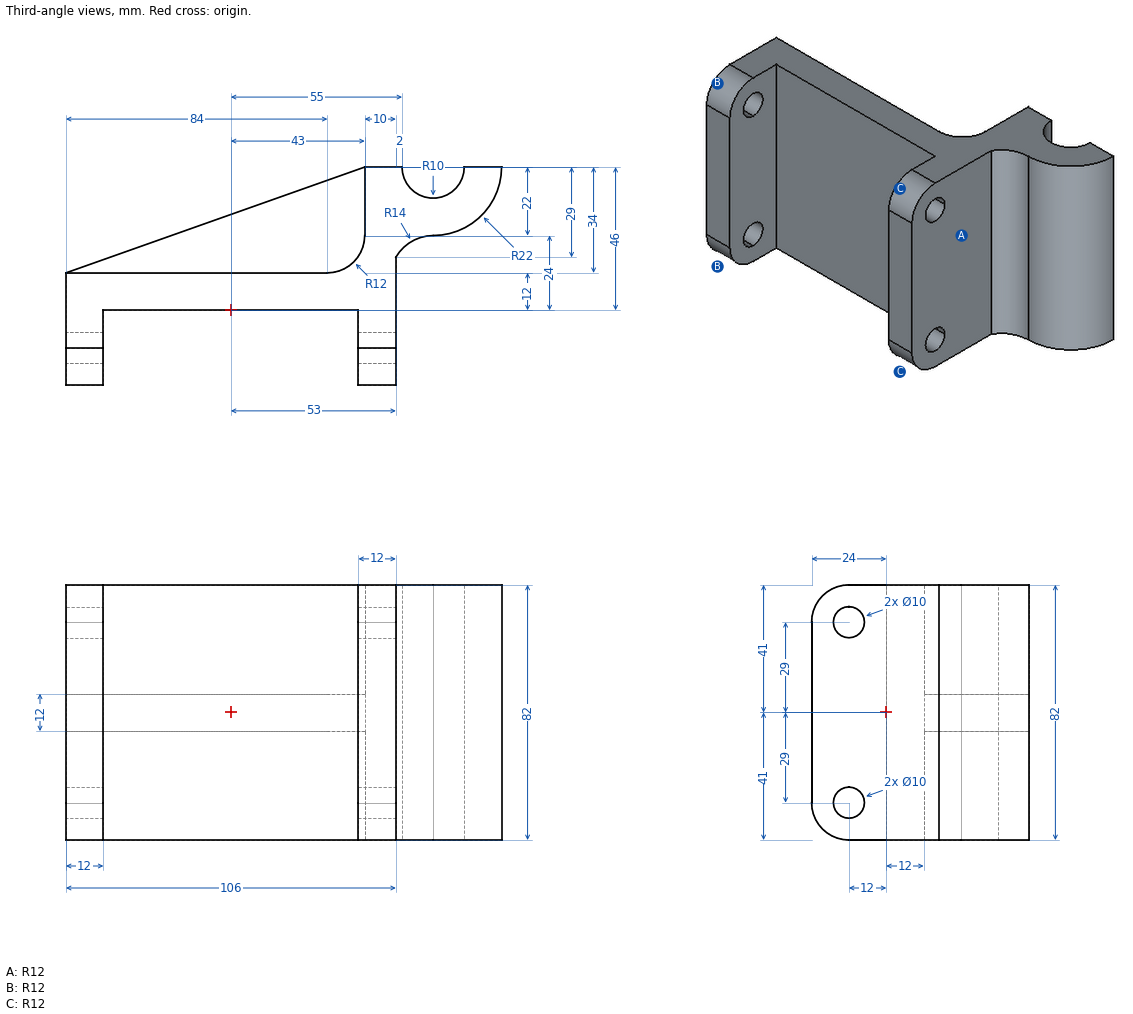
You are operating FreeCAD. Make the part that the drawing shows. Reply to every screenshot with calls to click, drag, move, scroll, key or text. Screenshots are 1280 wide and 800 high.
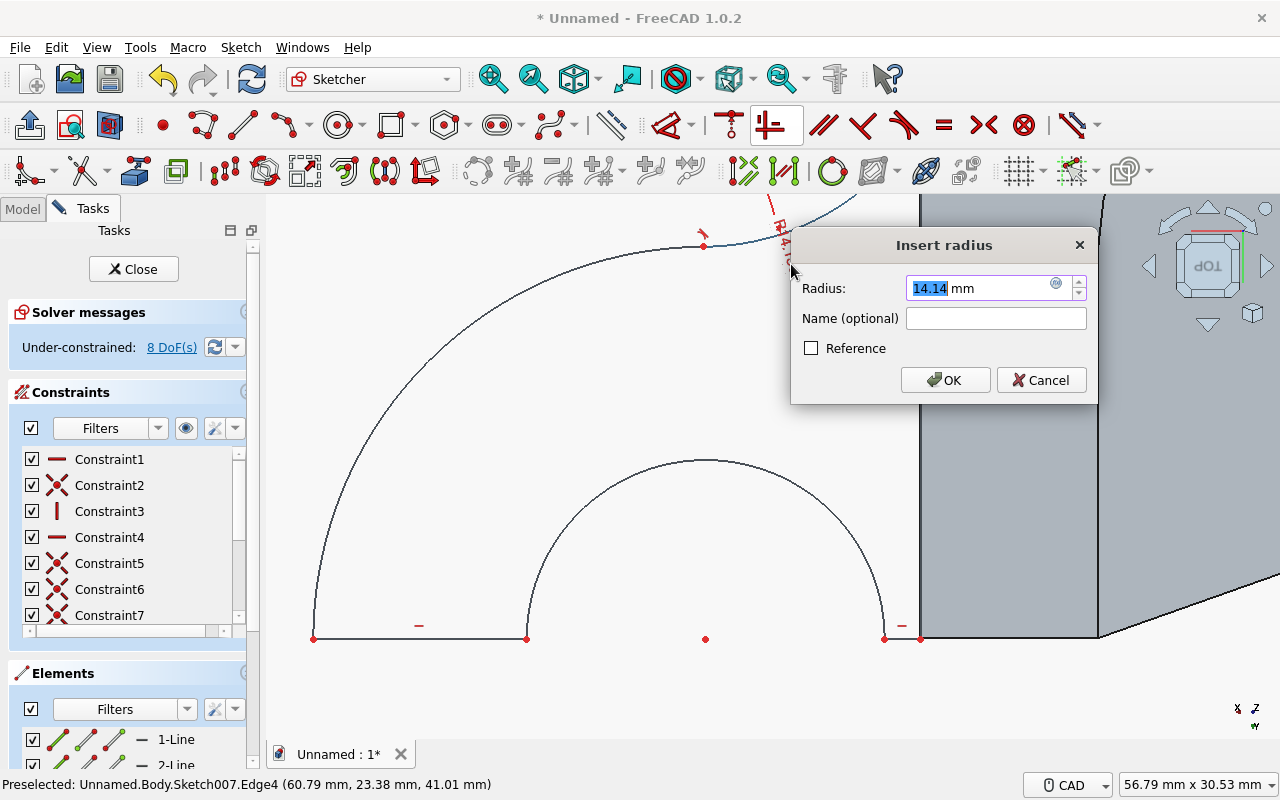
text(14)
key(Return)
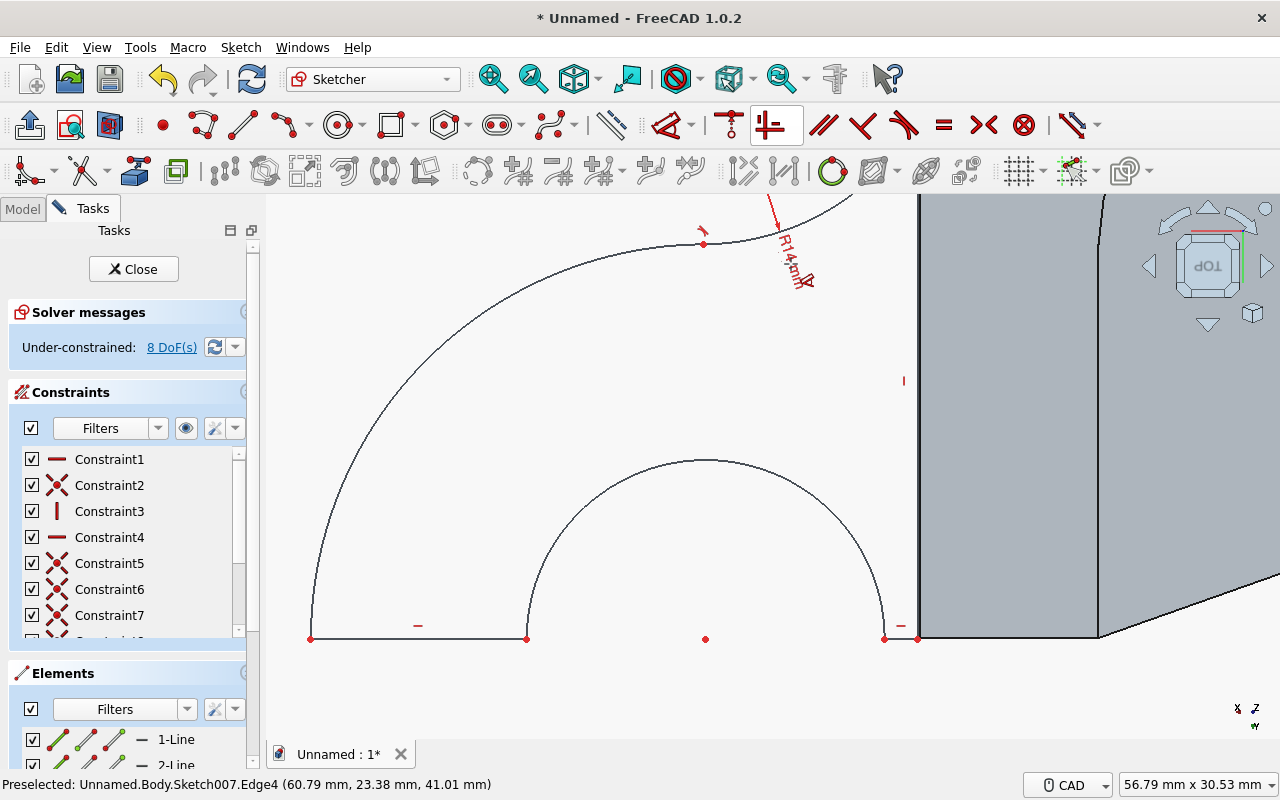
click(525, 288)
click(510, 260)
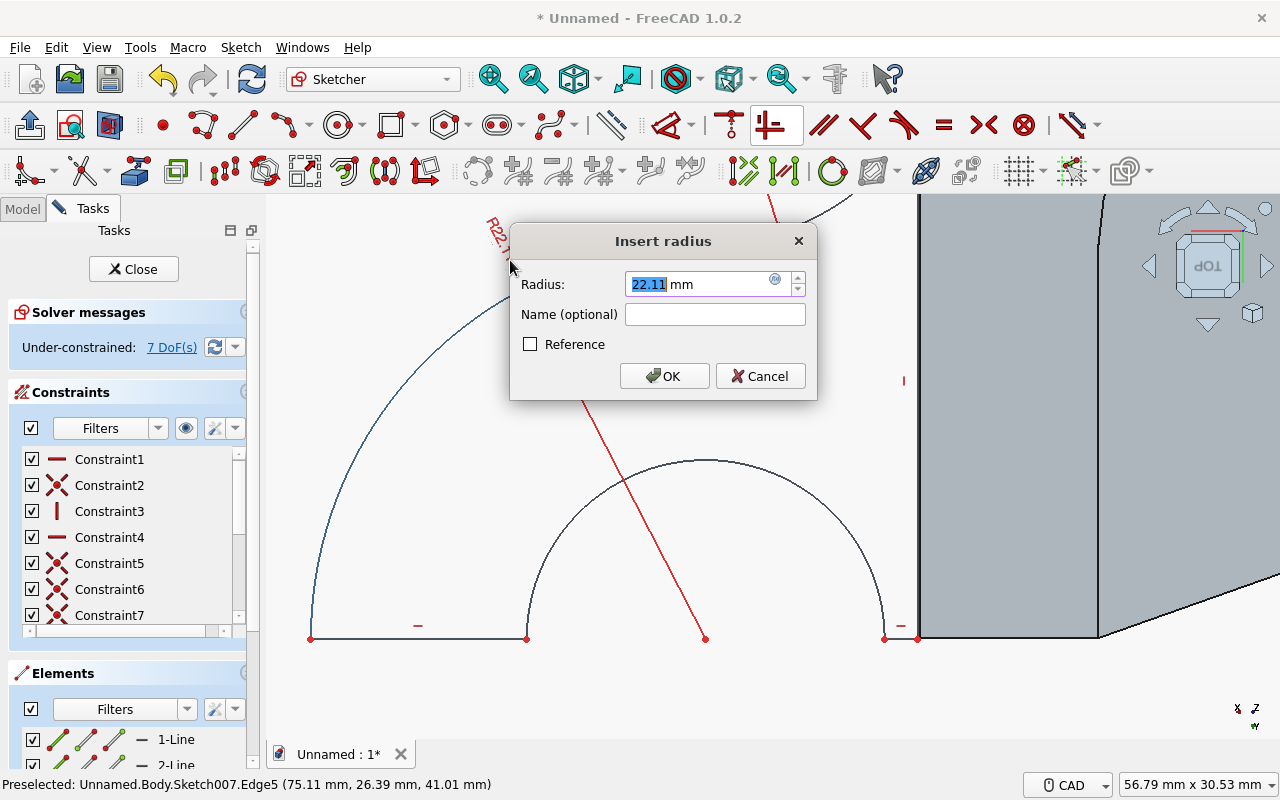
text(22)
key(Return)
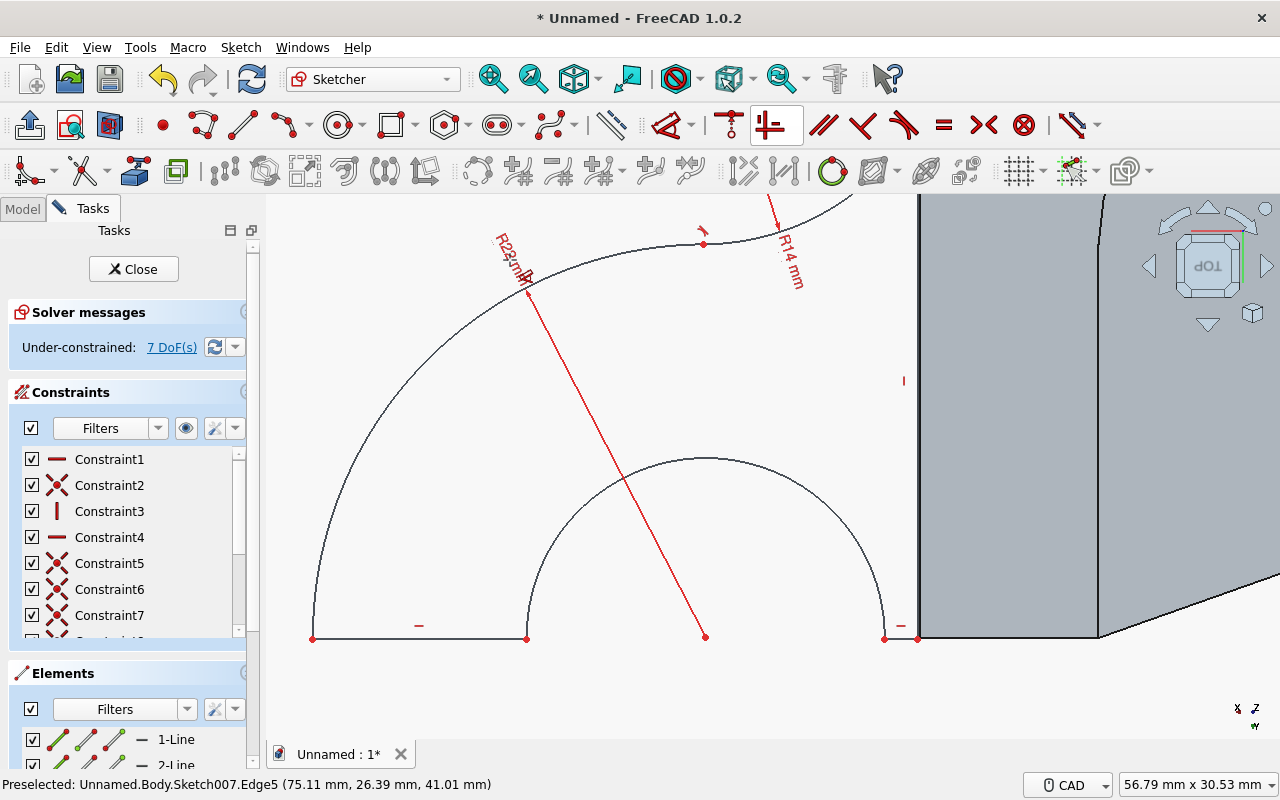
click(812, 493)
click(831, 467)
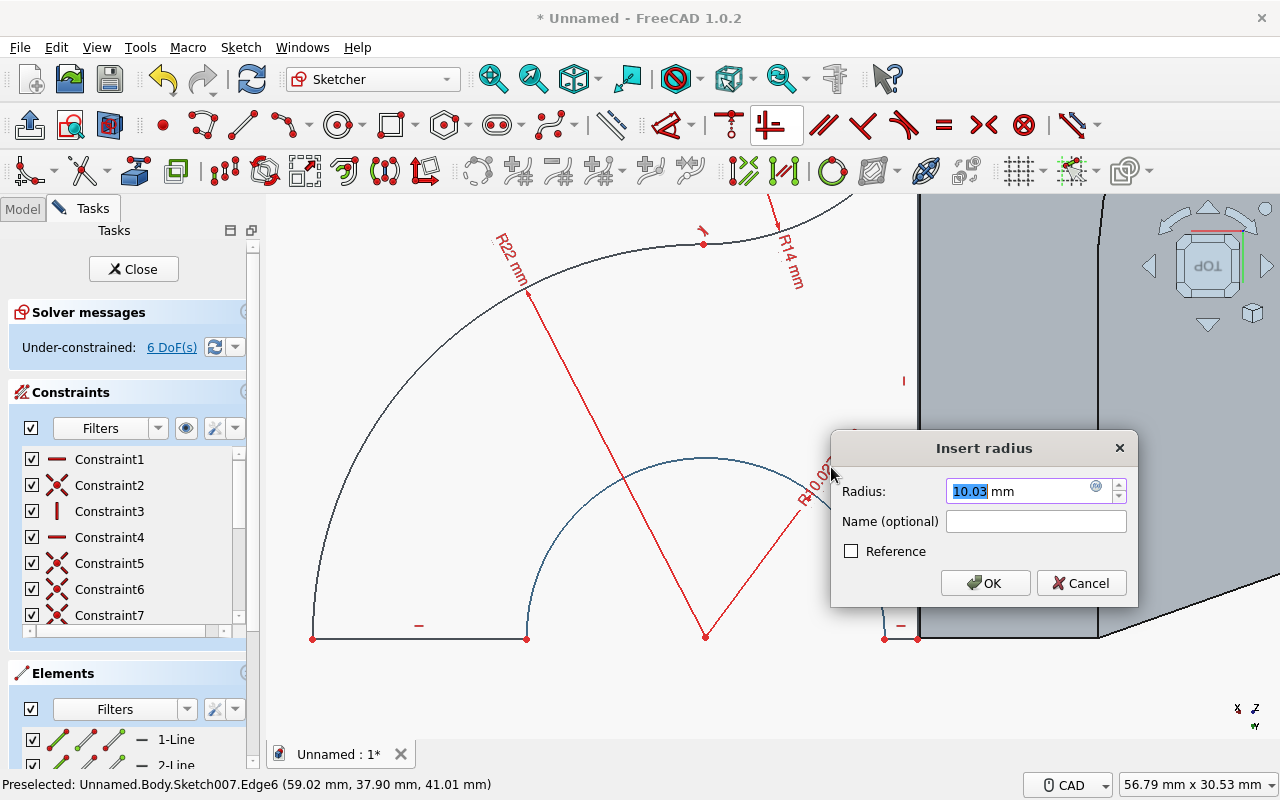
text(10)
key(Return)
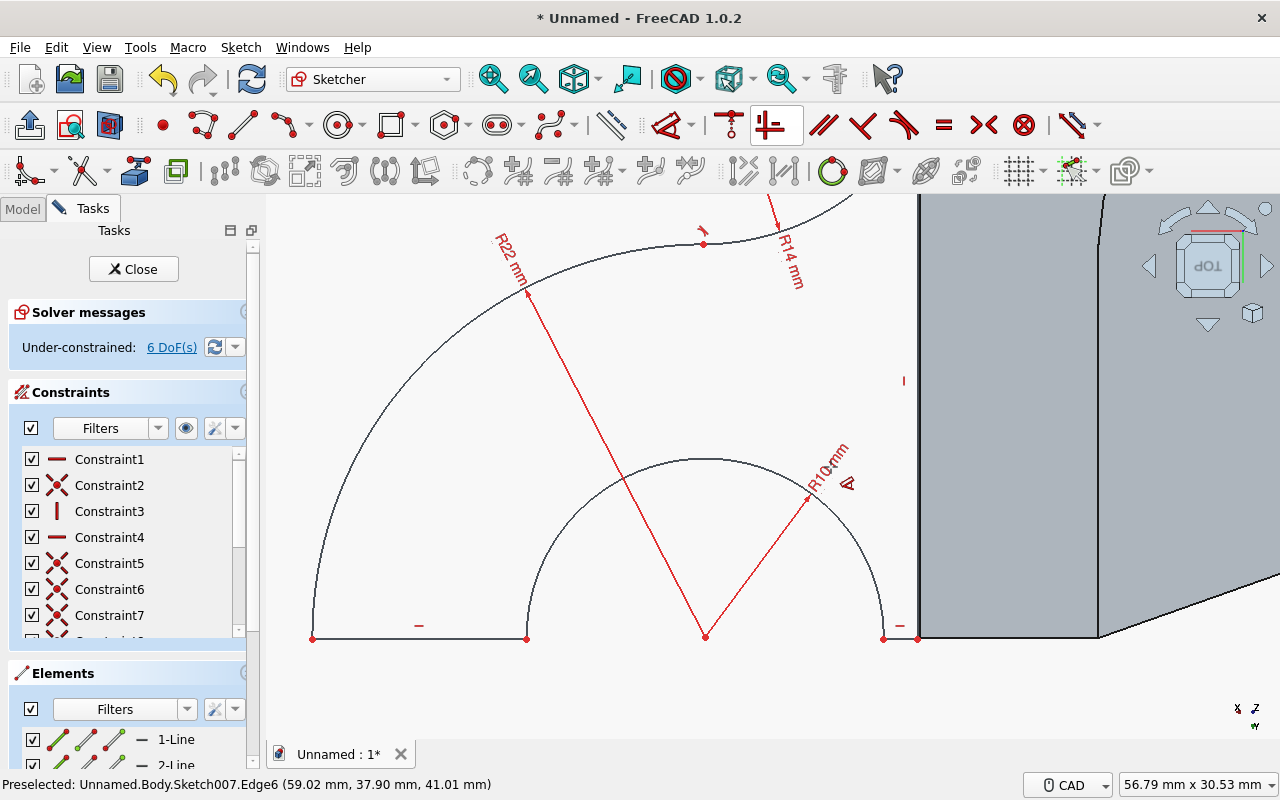
scroll(894, 639, up, 2)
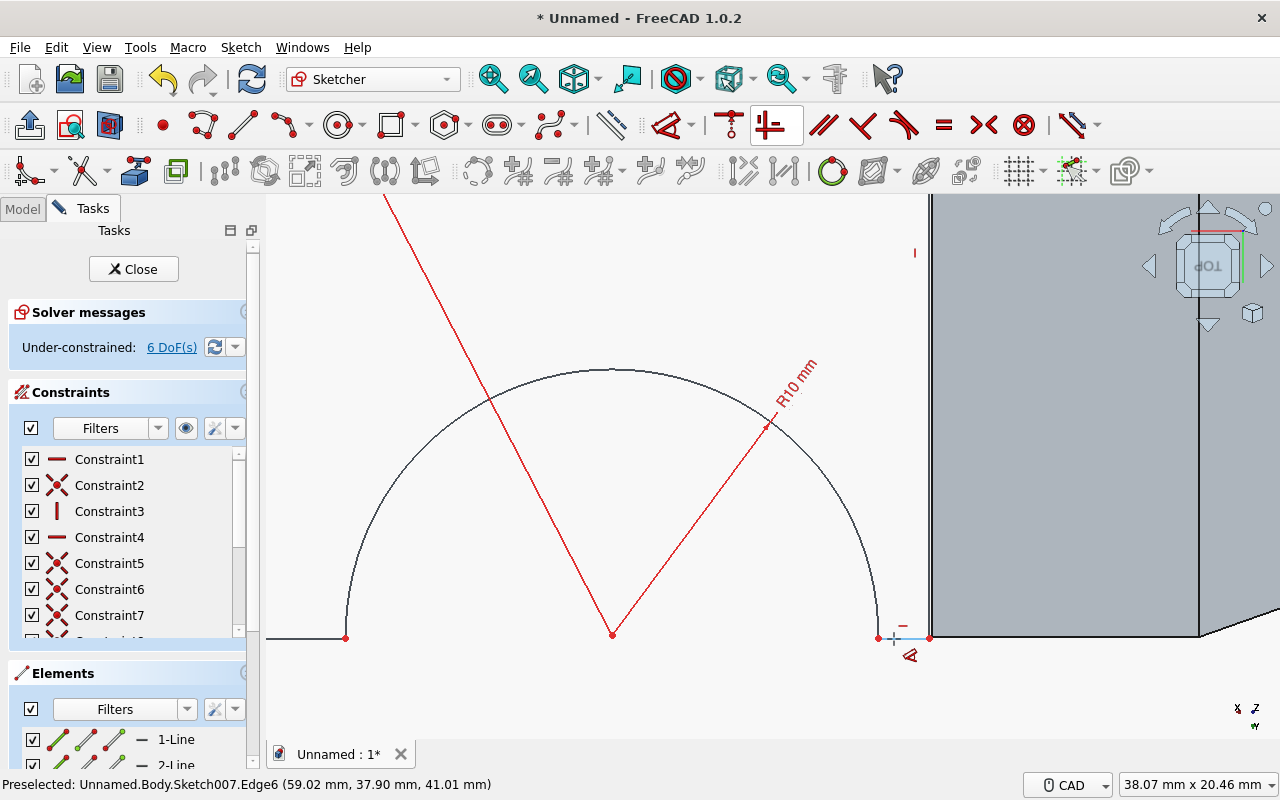
click(894, 639)
click(904, 673)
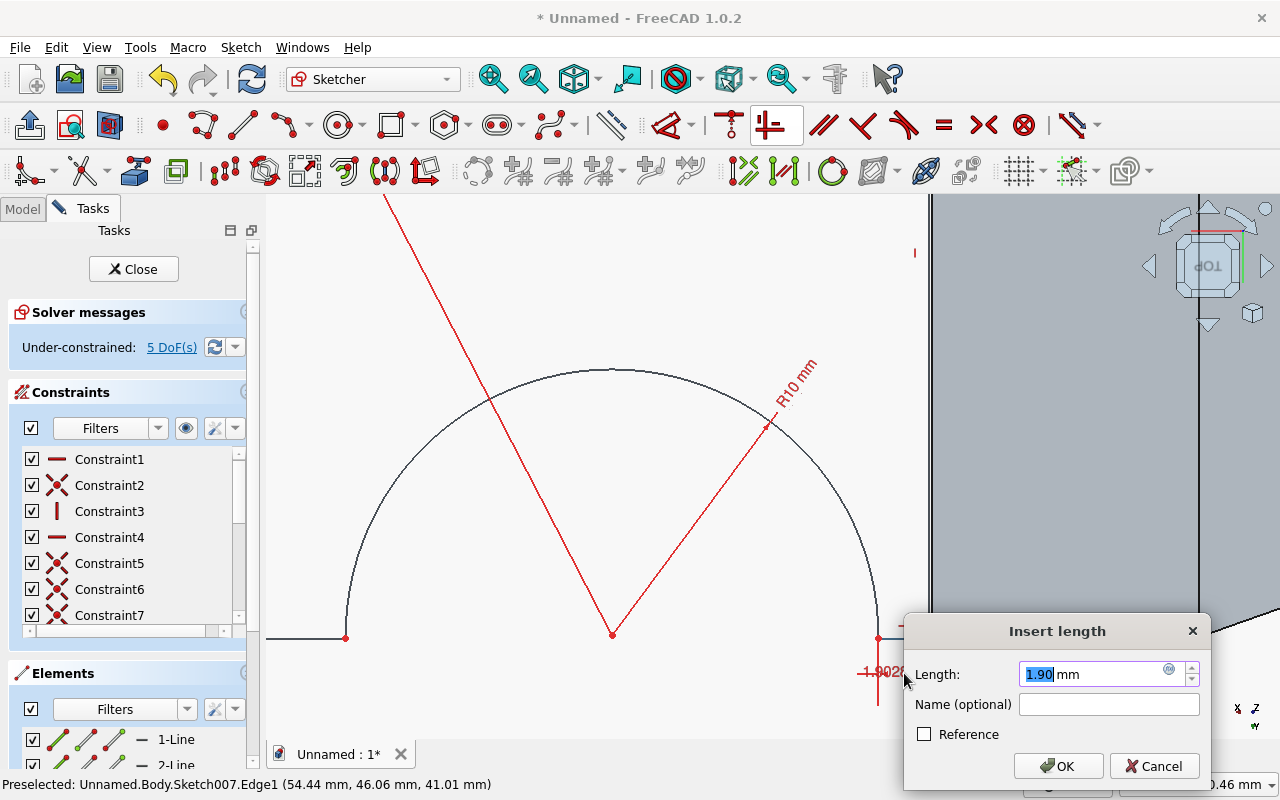
text(2)
key(Return)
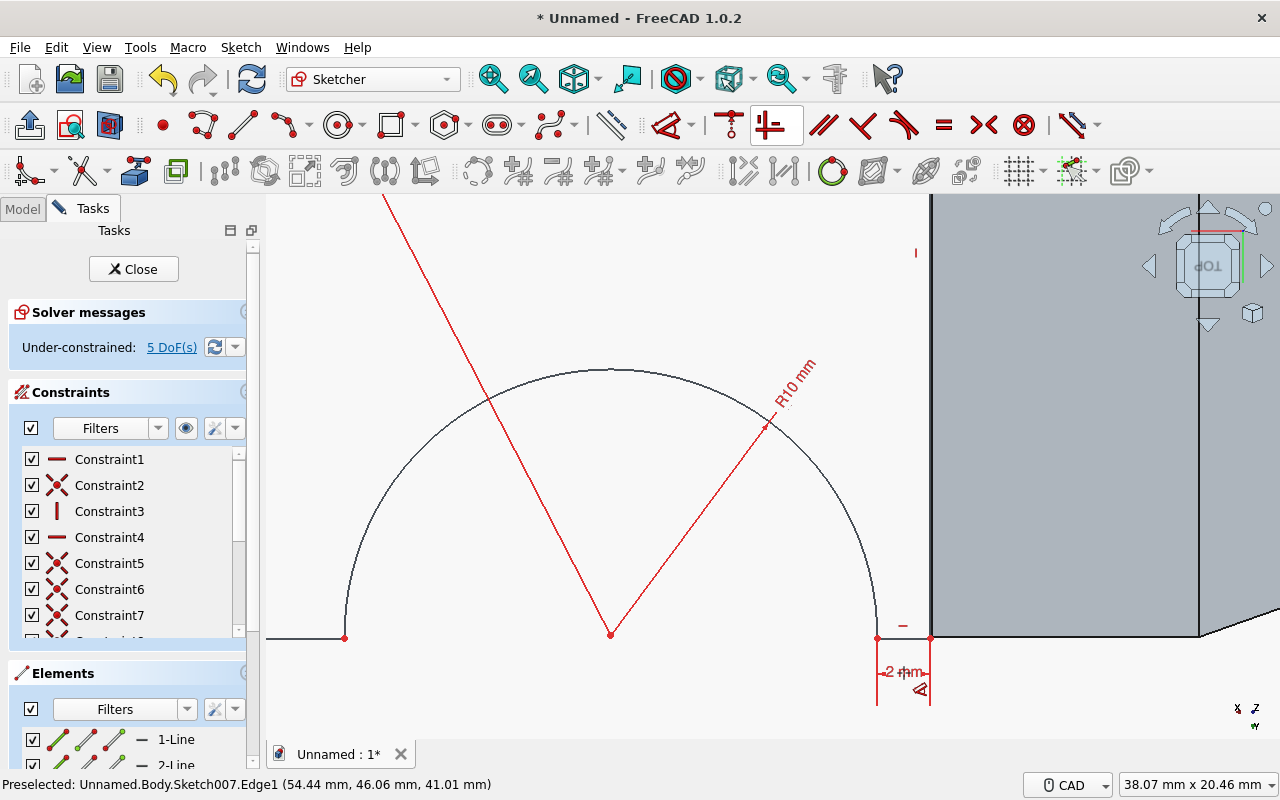
click(930, 407)
click(964, 430)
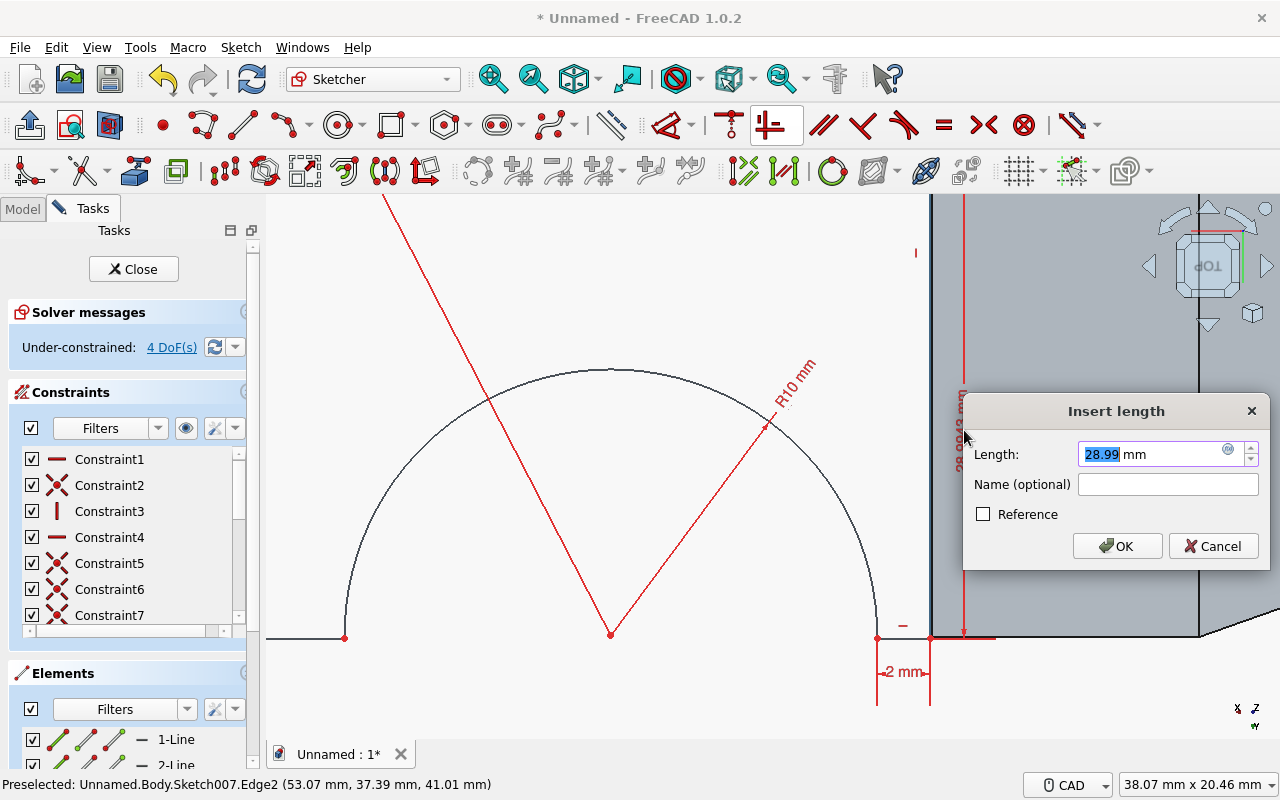
text(29)
key(Return)